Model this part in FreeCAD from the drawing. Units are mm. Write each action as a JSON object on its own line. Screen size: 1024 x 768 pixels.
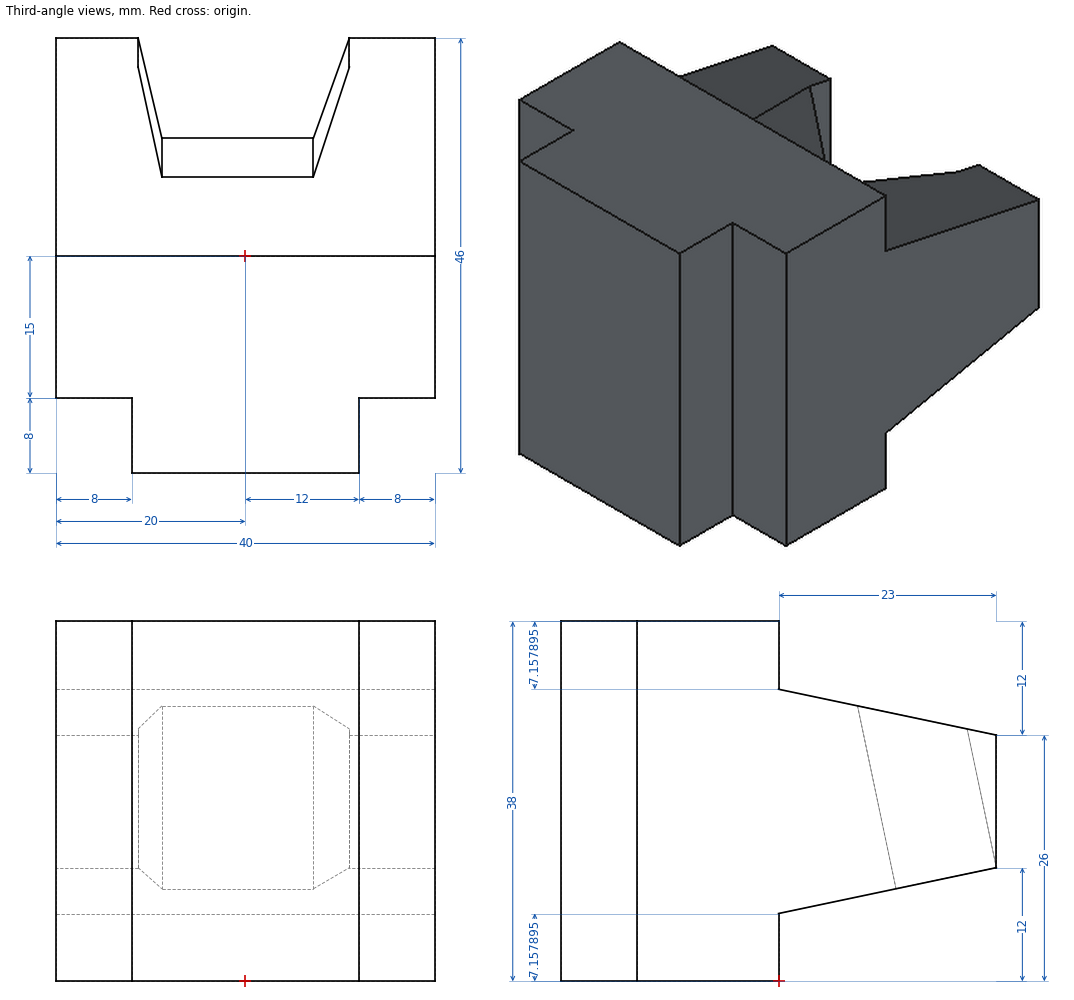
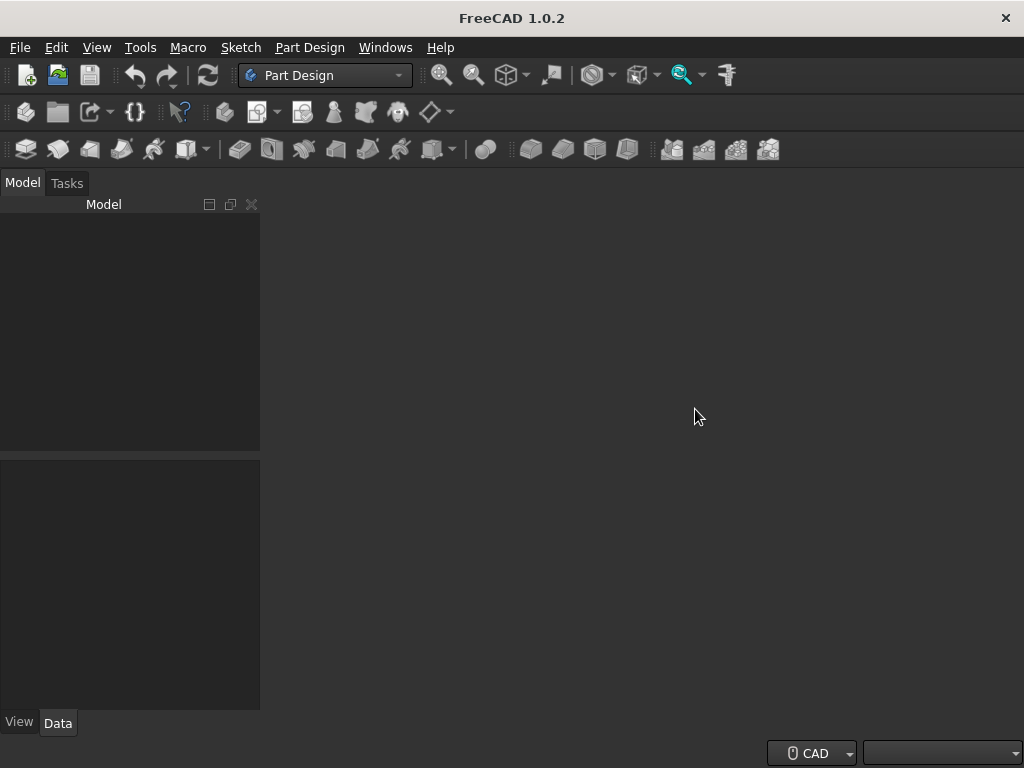
{"action": "left_click", "coordinate": [26, 76]}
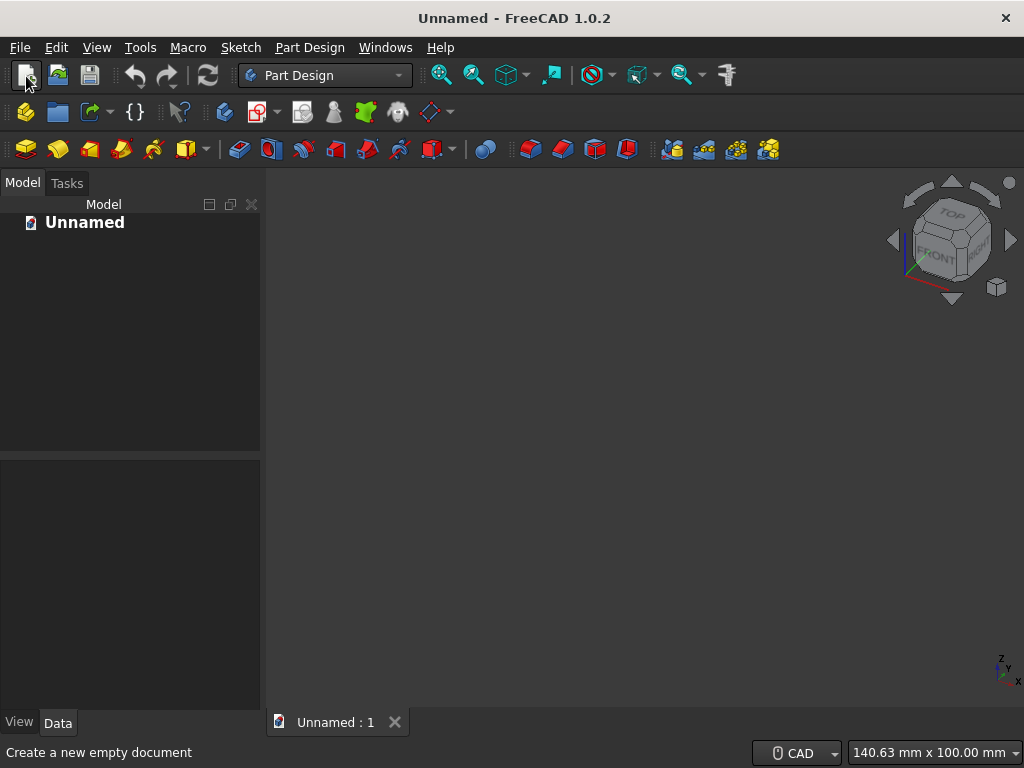
{"action": "left_click", "coordinate": [258, 112]}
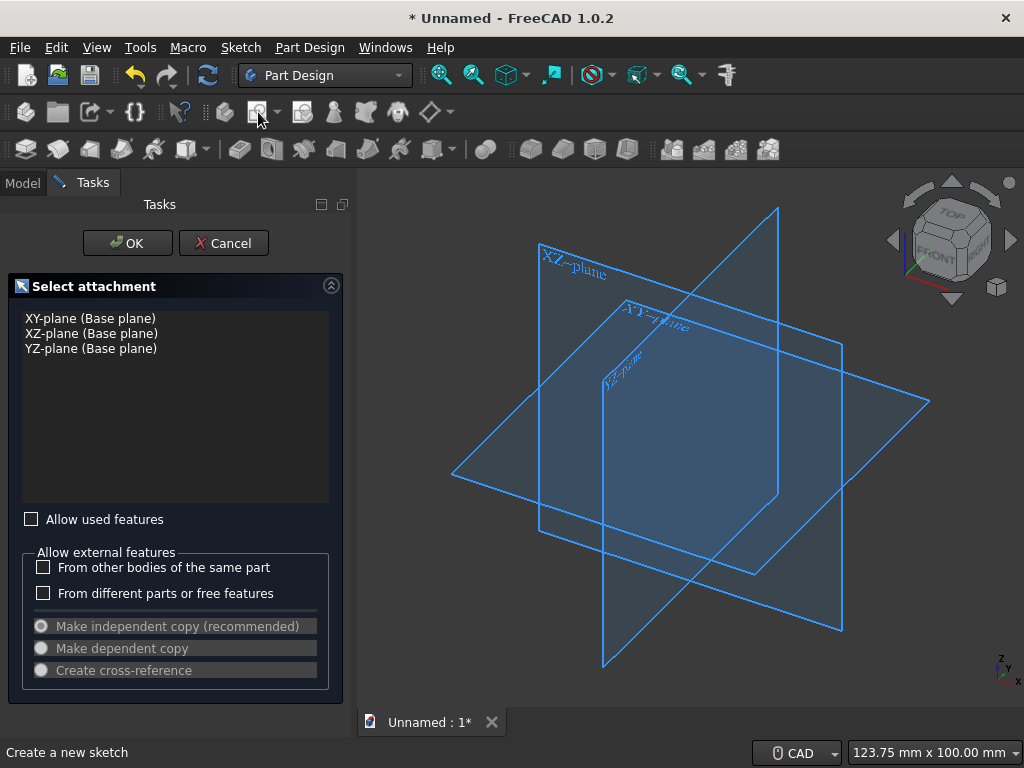
{"action": "left_click", "coordinate": [82, 318]}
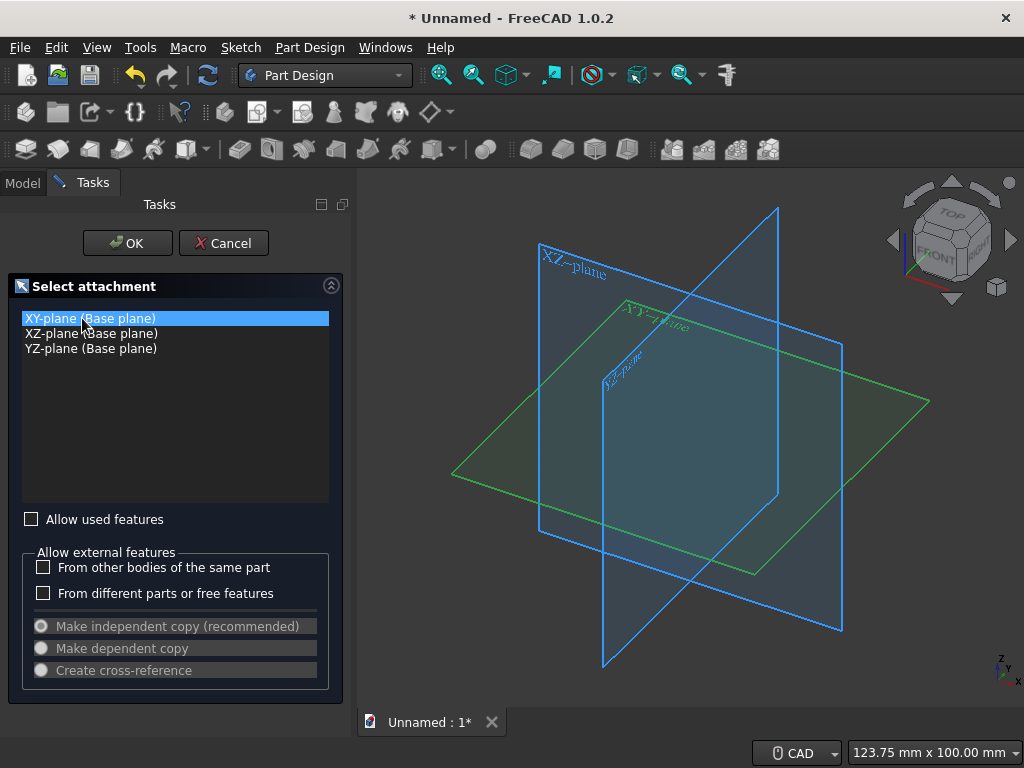
{"action": "left_click", "coordinate": [128, 243]}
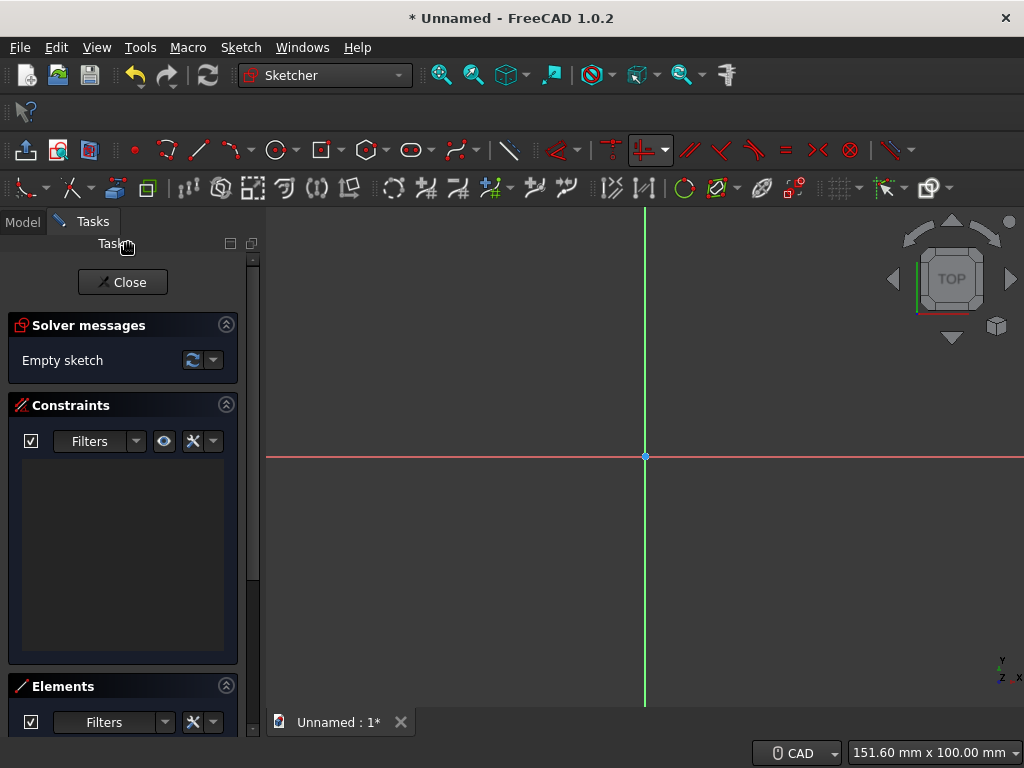
{"action": "scroll", "coordinate": [784, 457], "scroll_direction": "up", "scroll_amount": 2}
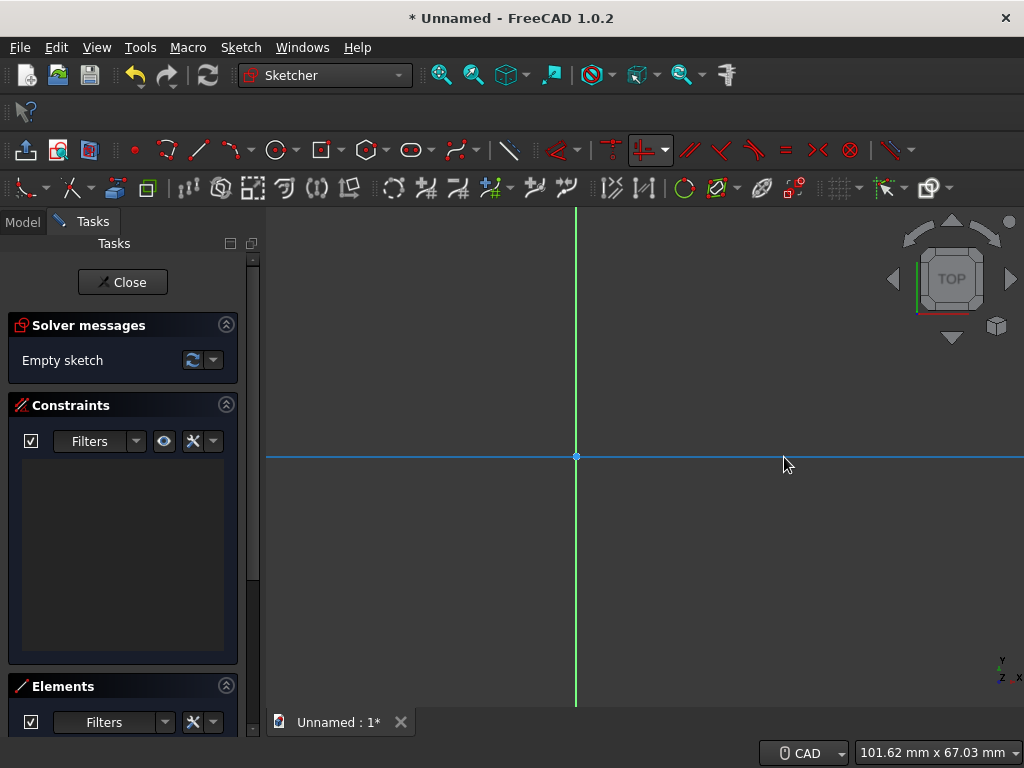
{"action": "left_click", "coordinate": [322, 150]}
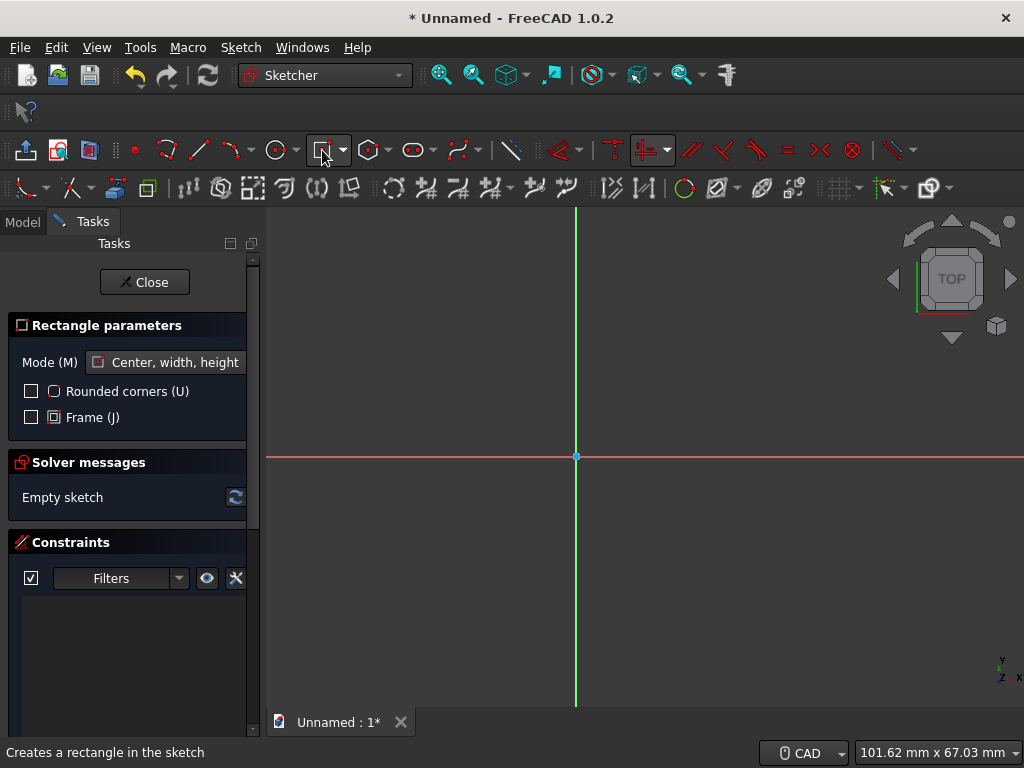
{"action": "left_click", "coordinate": [576, 457]}
{"action": "left_click", "coordinate": [725, 285]}
{"action": "key", "text": "Escape"}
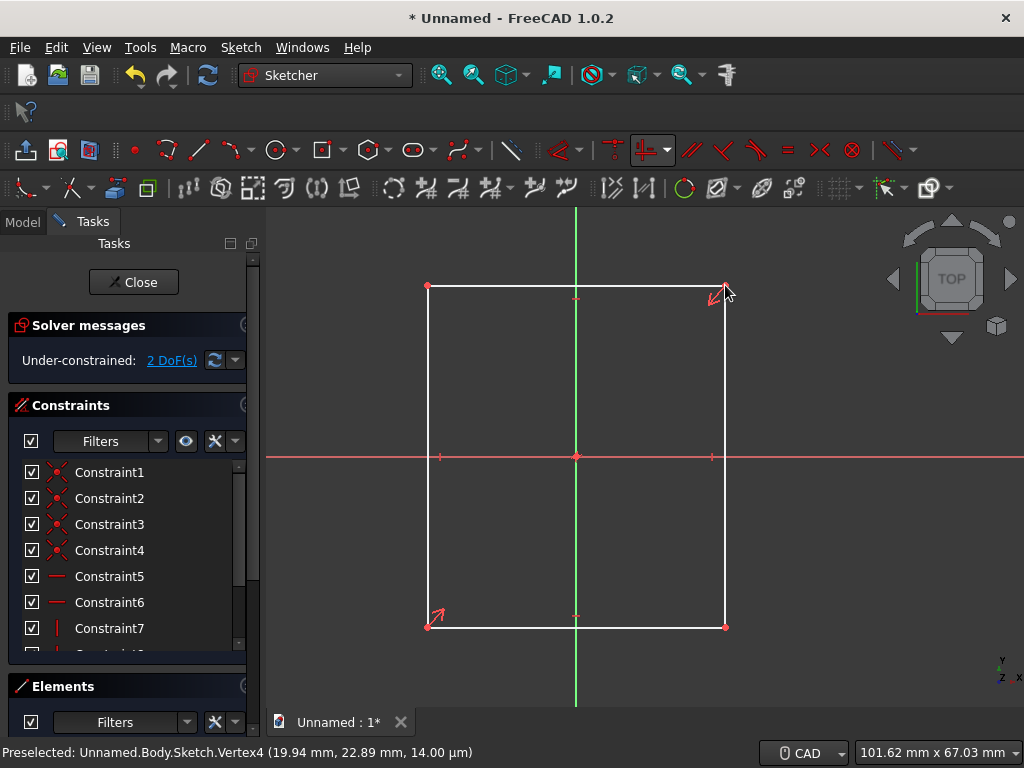
{"action": "left_click", "coordinate": [517, 628]}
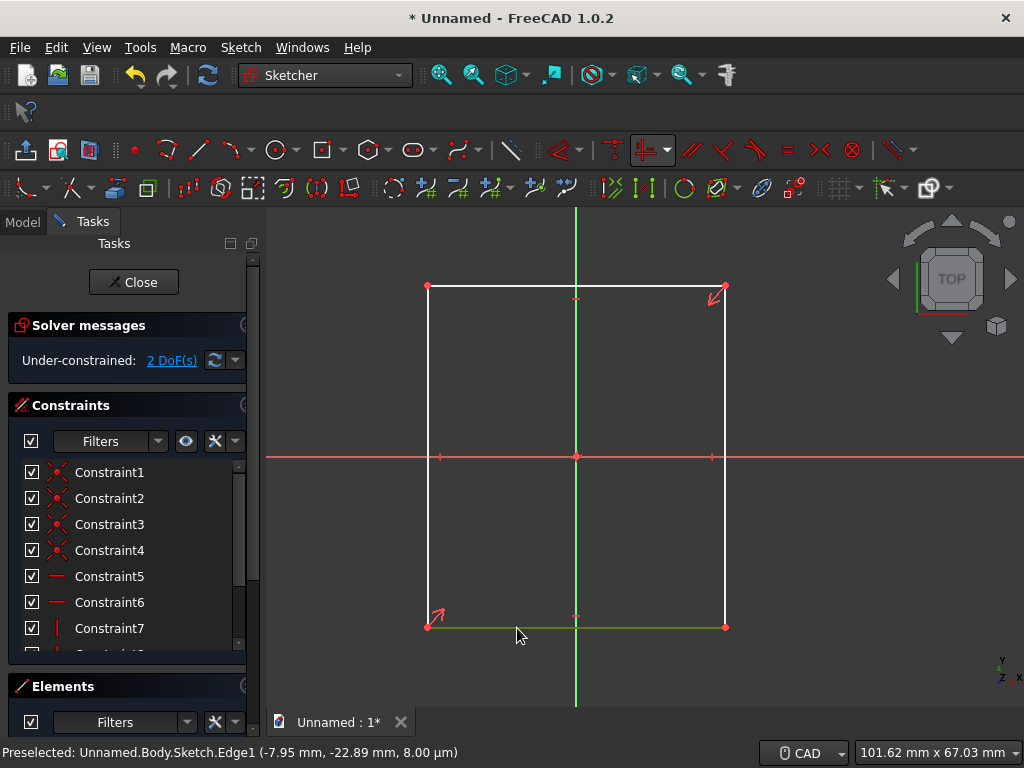
{"action": "left_click", "coordinate": [582, 150]}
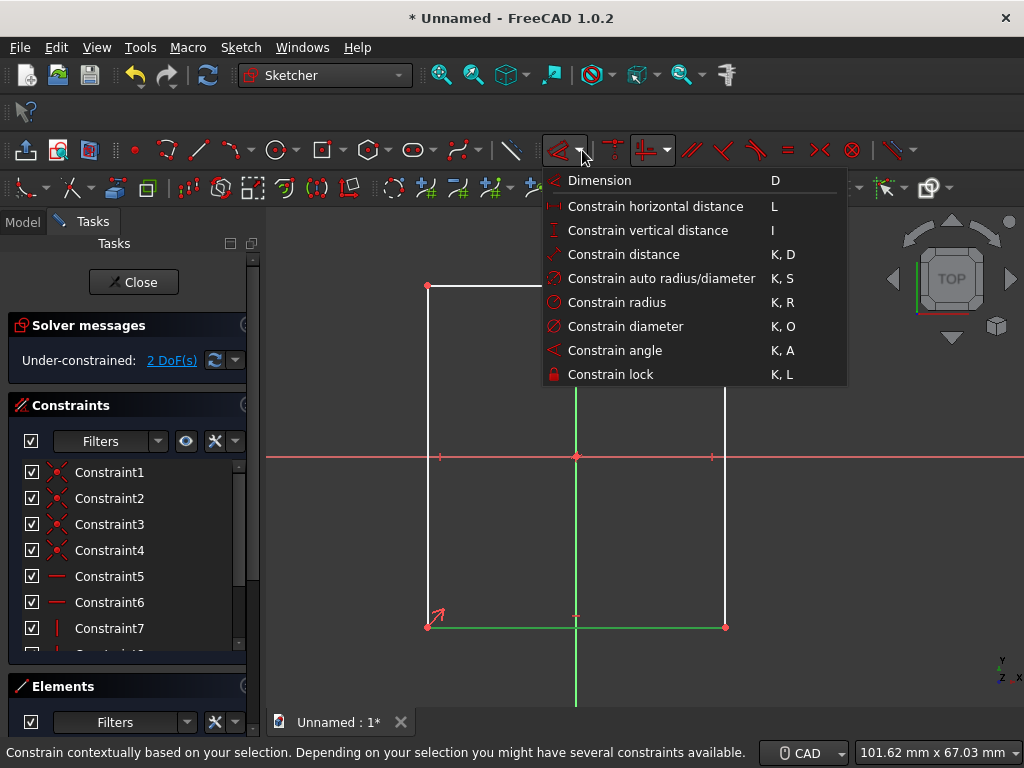
{"action": "left_click", "coordinate": [695, 206]}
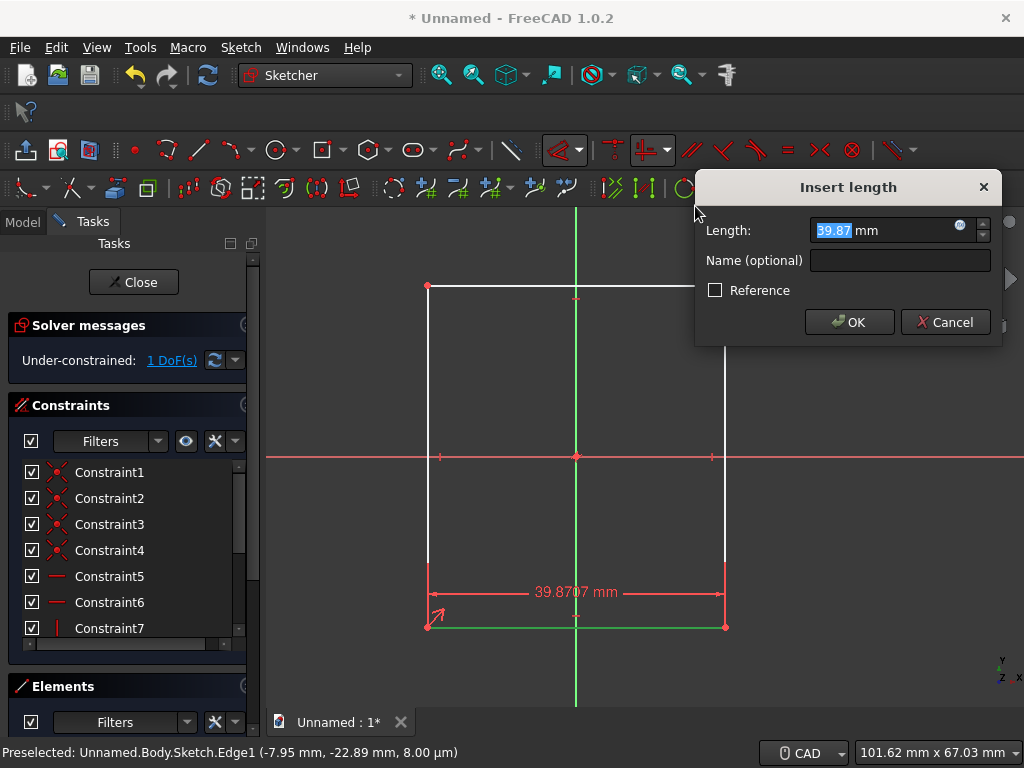
{"action": "type", "text": "40"}
{"action": "key", "text": "Return"}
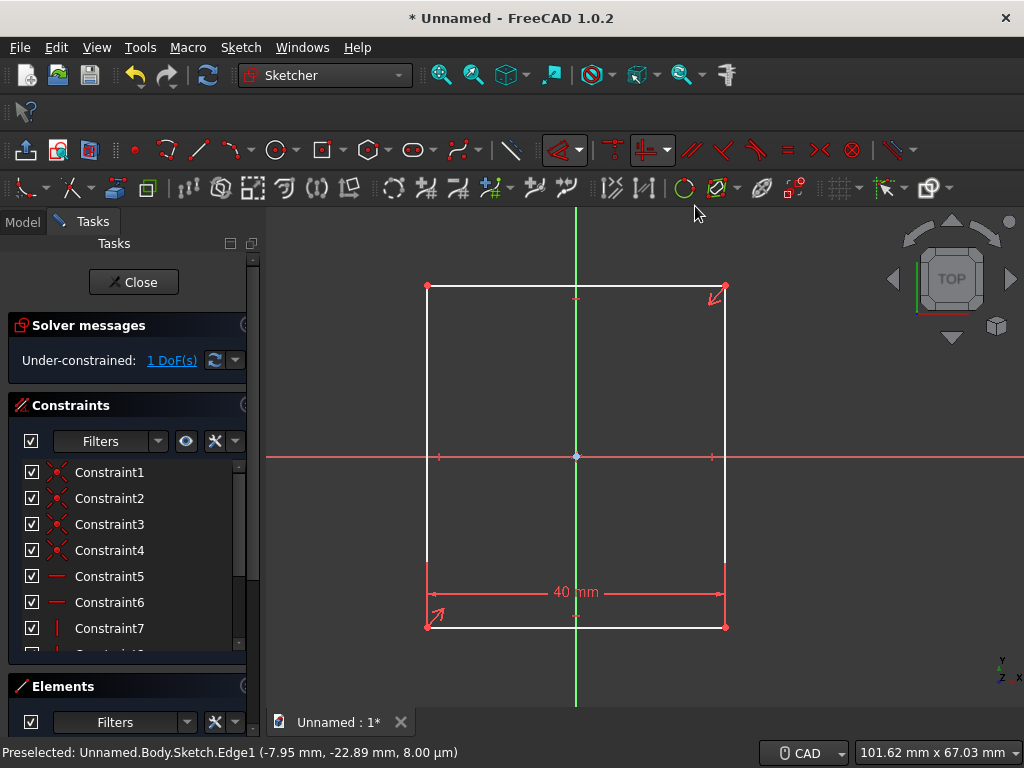
{"action": "left_click", "coordinate": [725, 525]}